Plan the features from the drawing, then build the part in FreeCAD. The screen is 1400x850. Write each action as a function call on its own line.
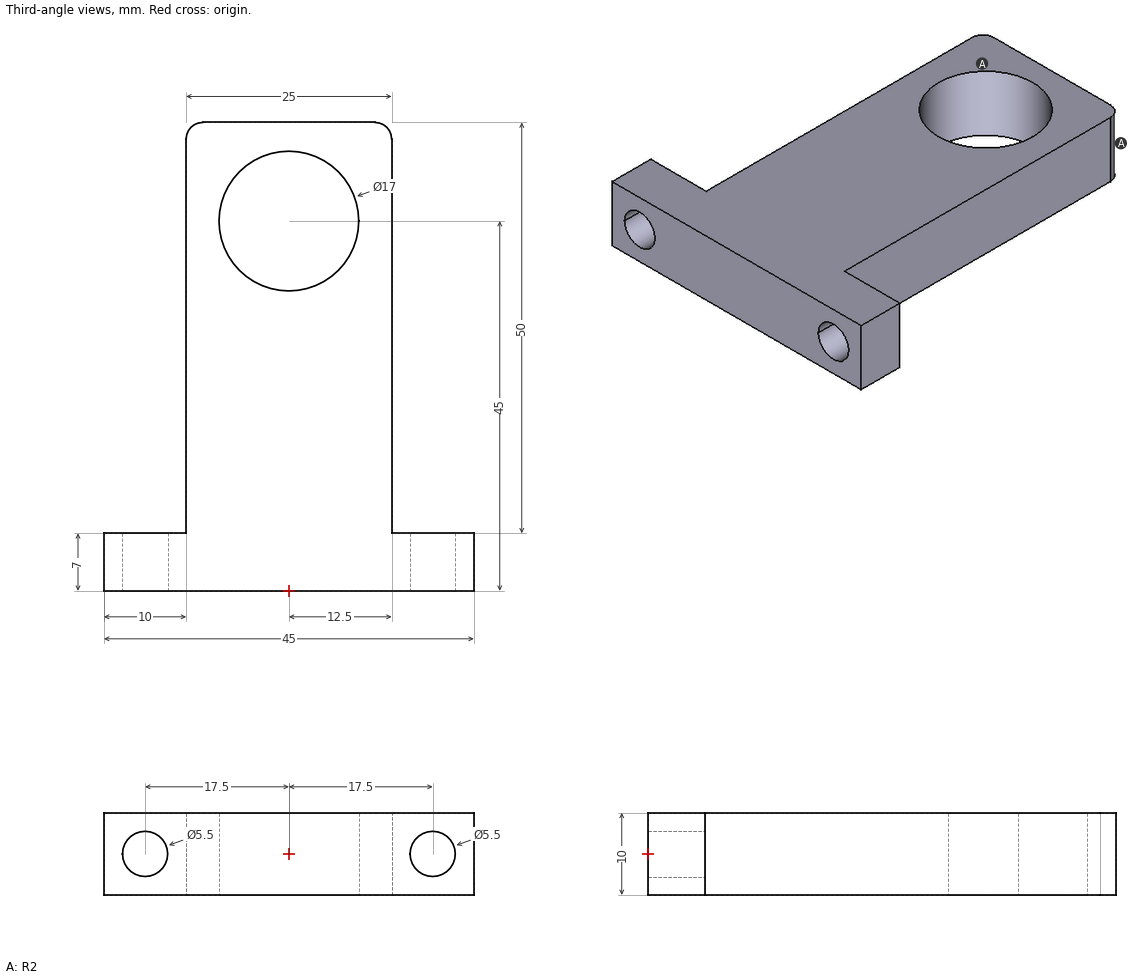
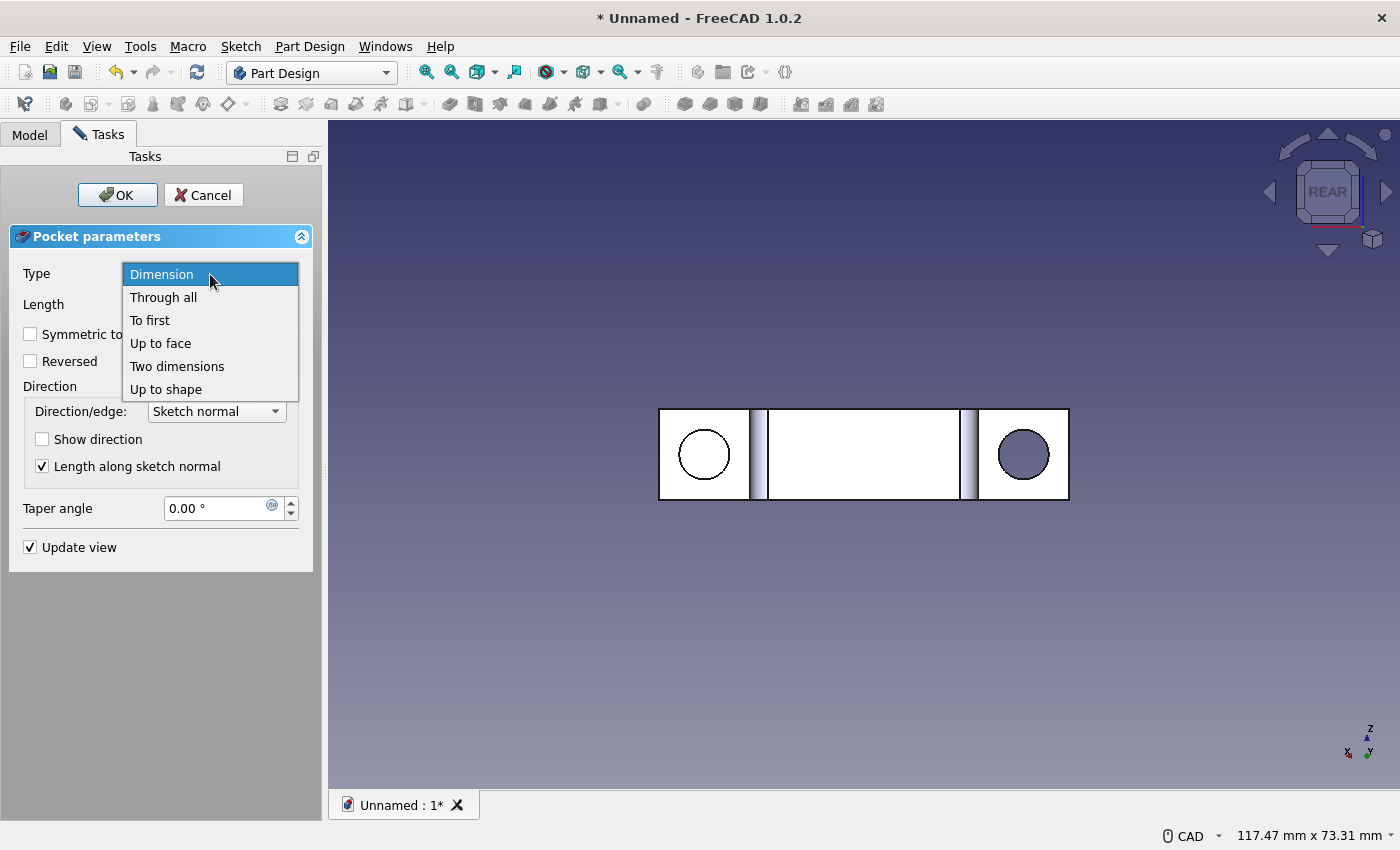
click(208, 320)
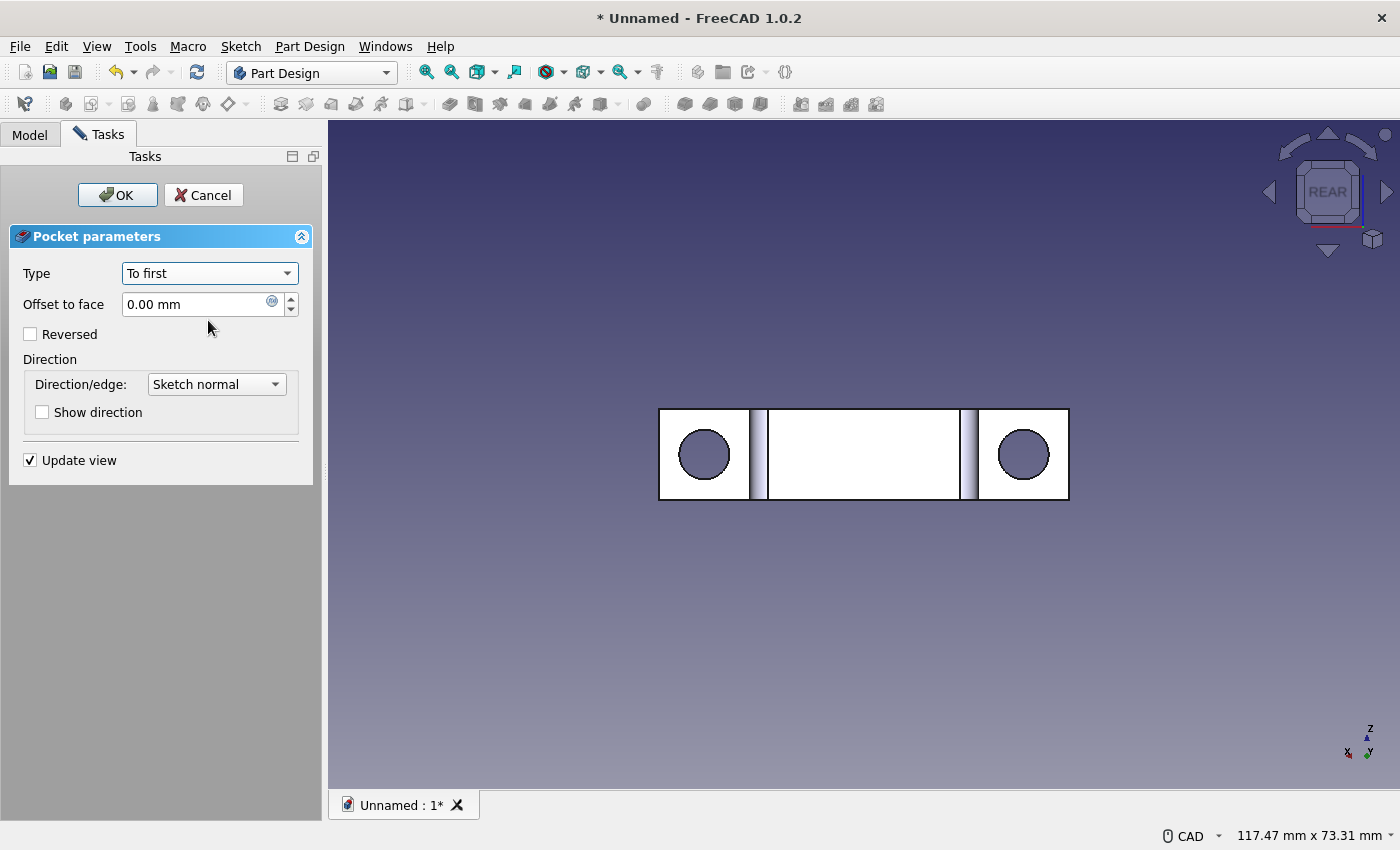
click(118, 195)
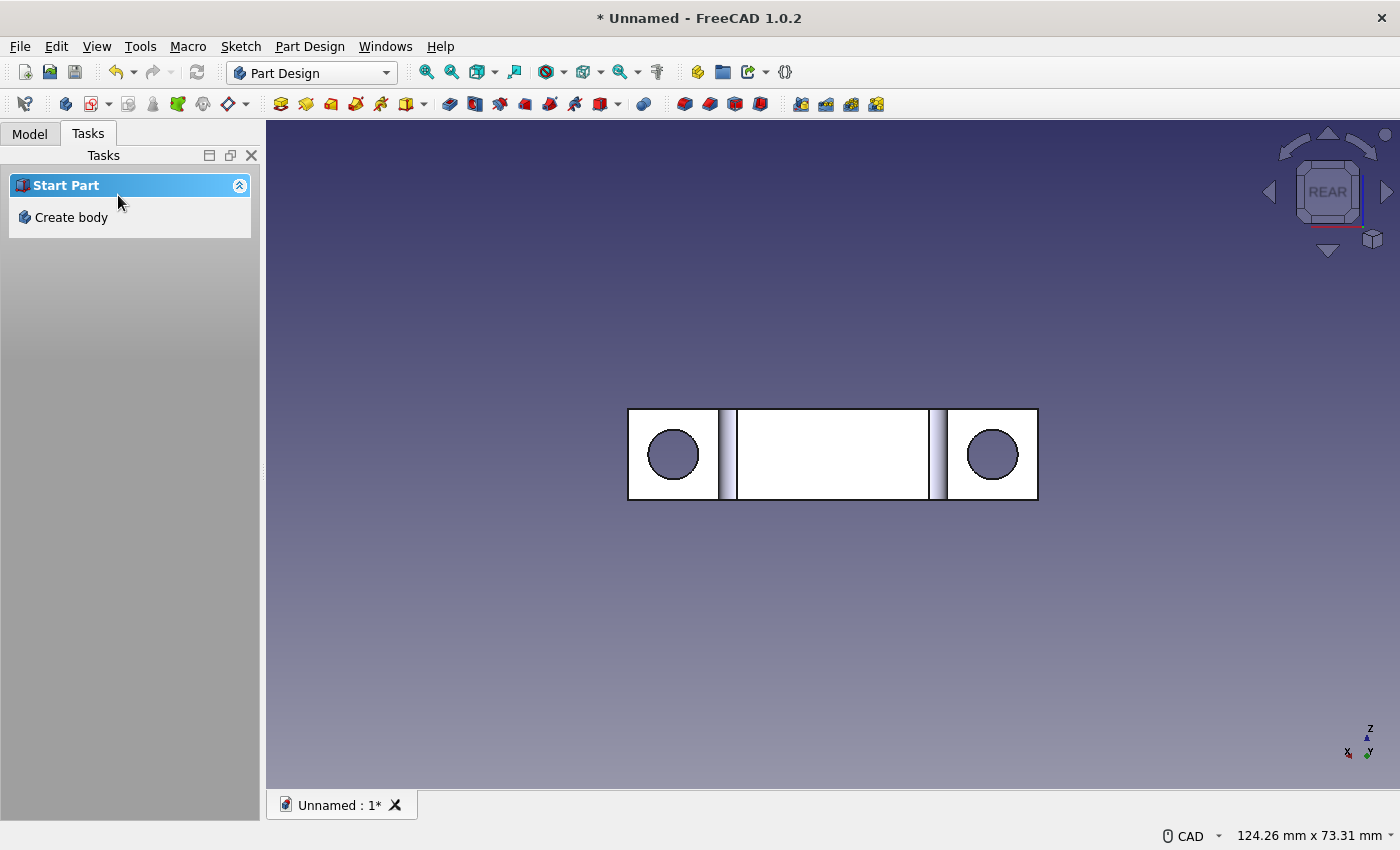
key(0)